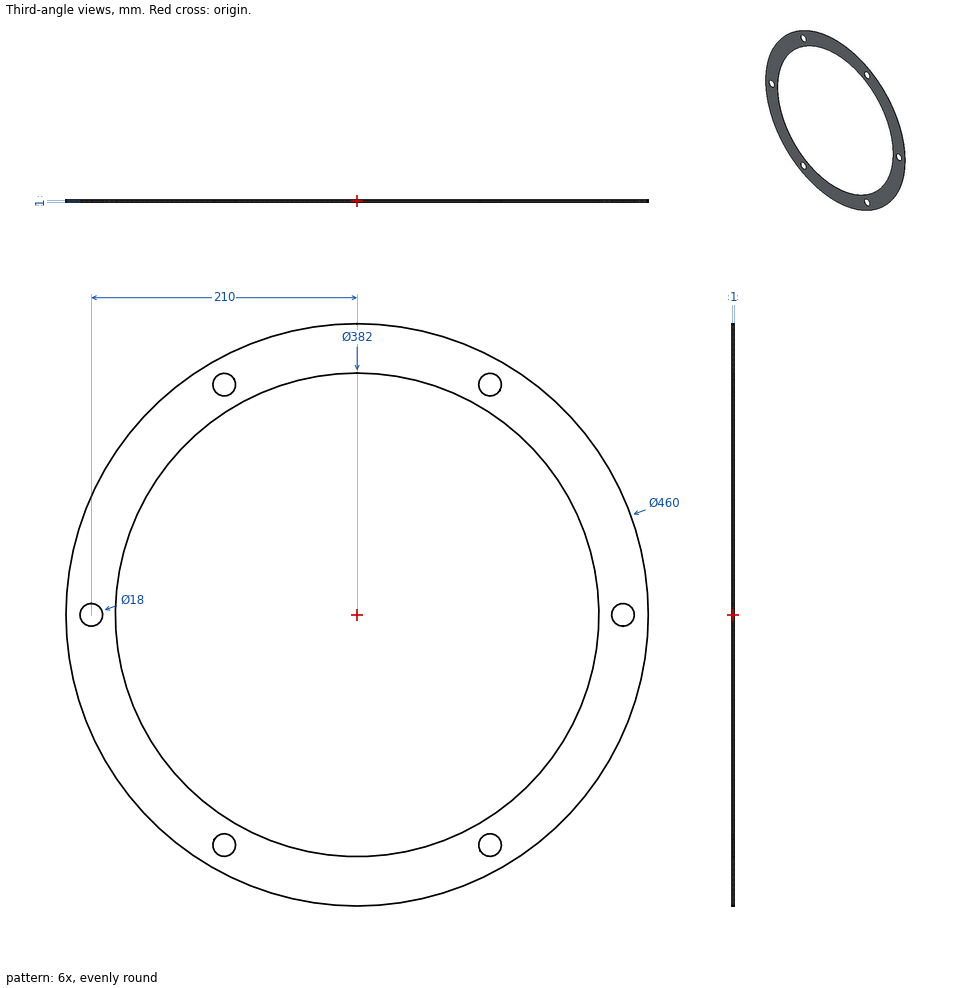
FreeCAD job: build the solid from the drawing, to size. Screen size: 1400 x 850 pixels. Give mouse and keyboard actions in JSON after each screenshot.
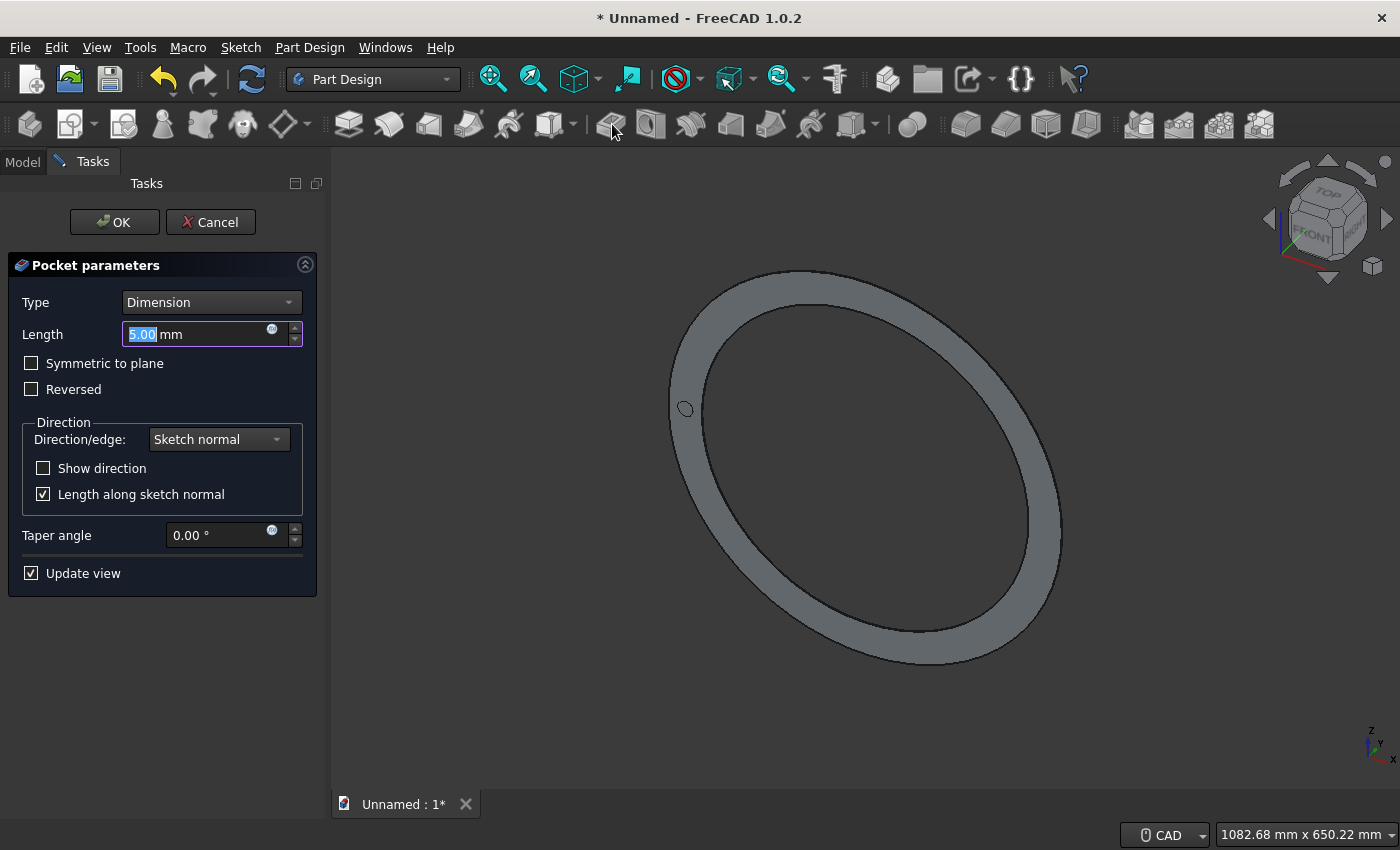
{"action": "type", "text": "1"}
{"action": "key", "text": "Tab"}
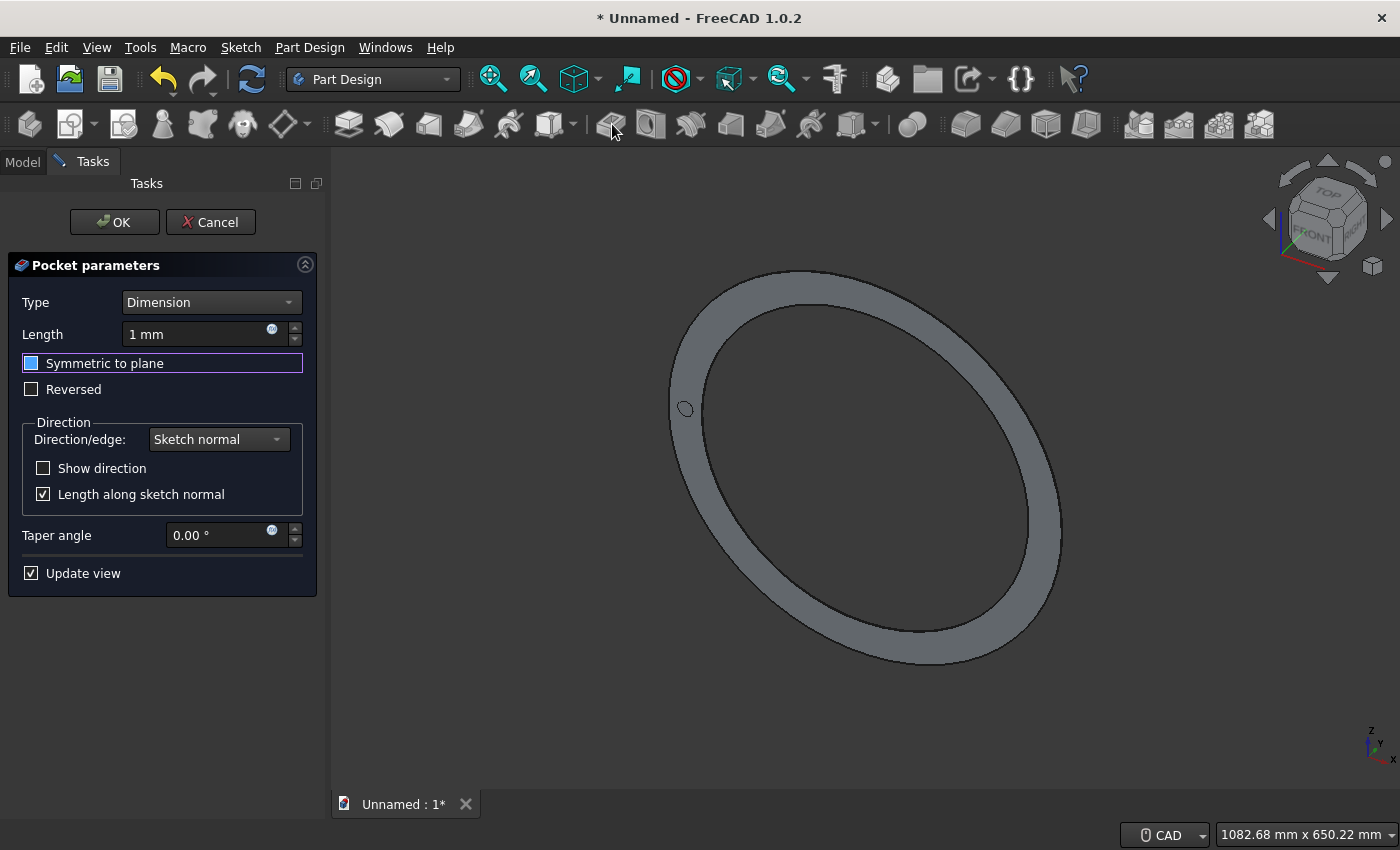
{"action": "left_click", "coordinate": [30, 363]}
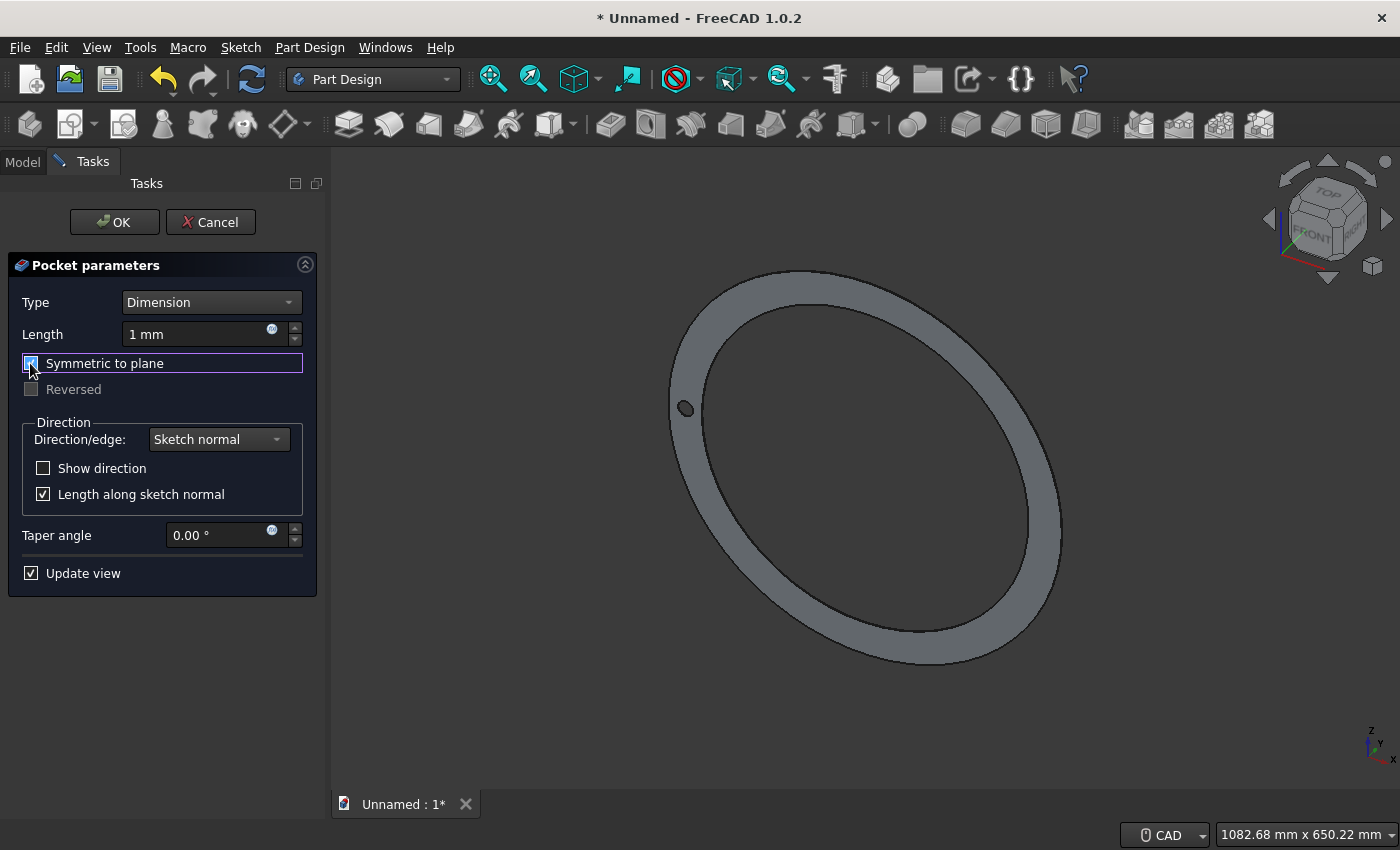
{"action": "left_click", "coordinate": [115, 222]}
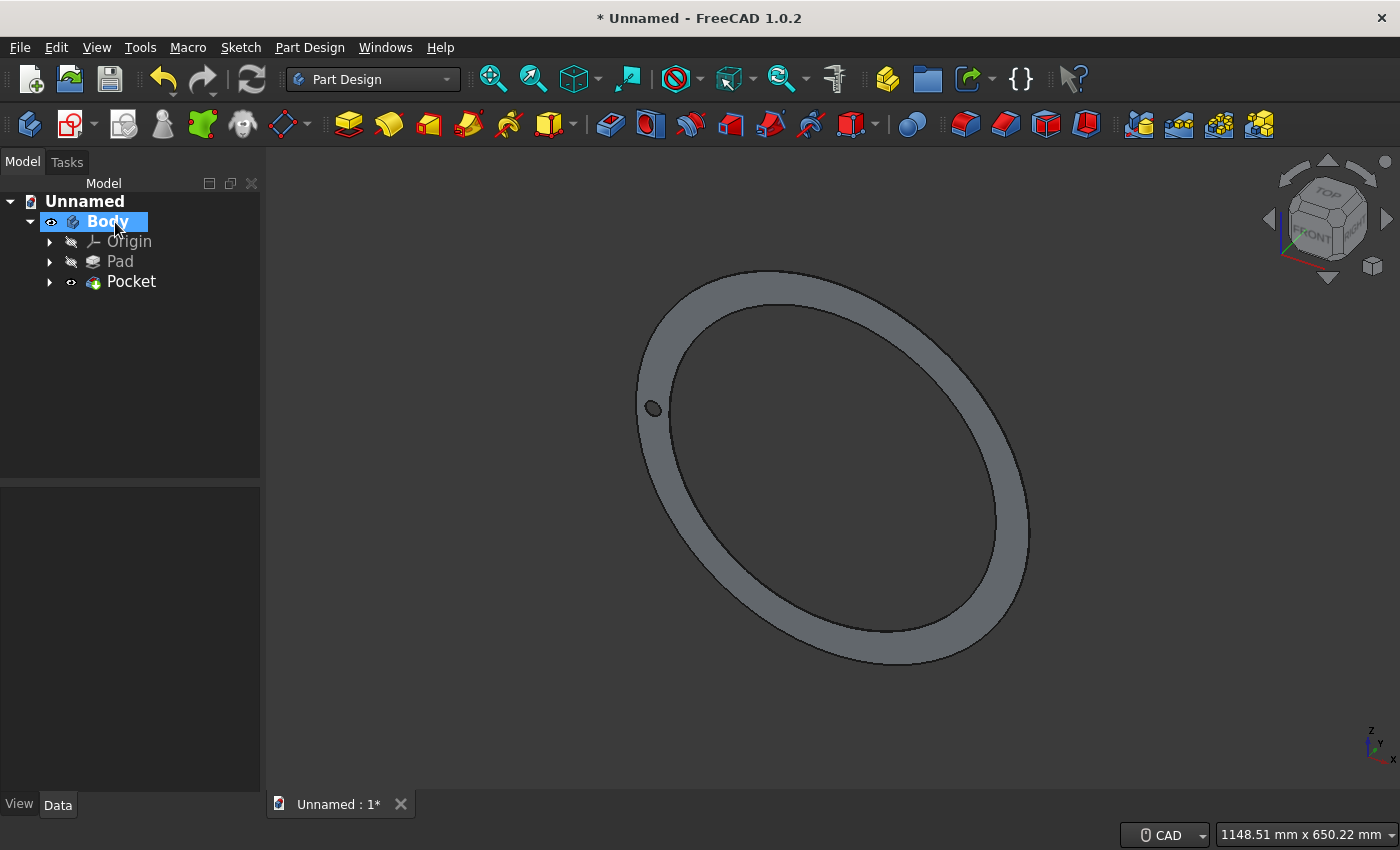
{"action": "left_click", "coordinate": [116, 282]}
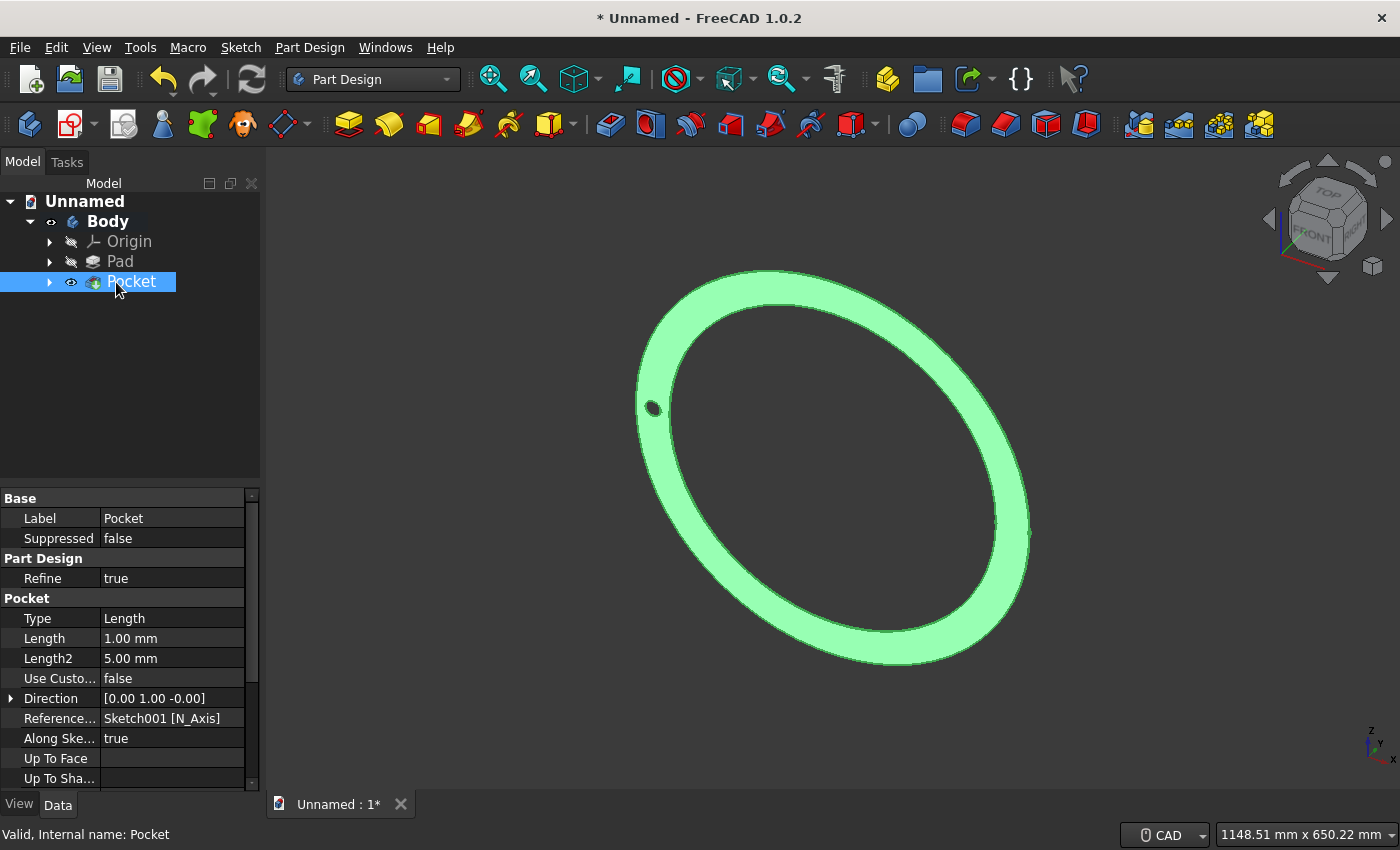
{"action": "left_click", "coordinate": [1220, 124]}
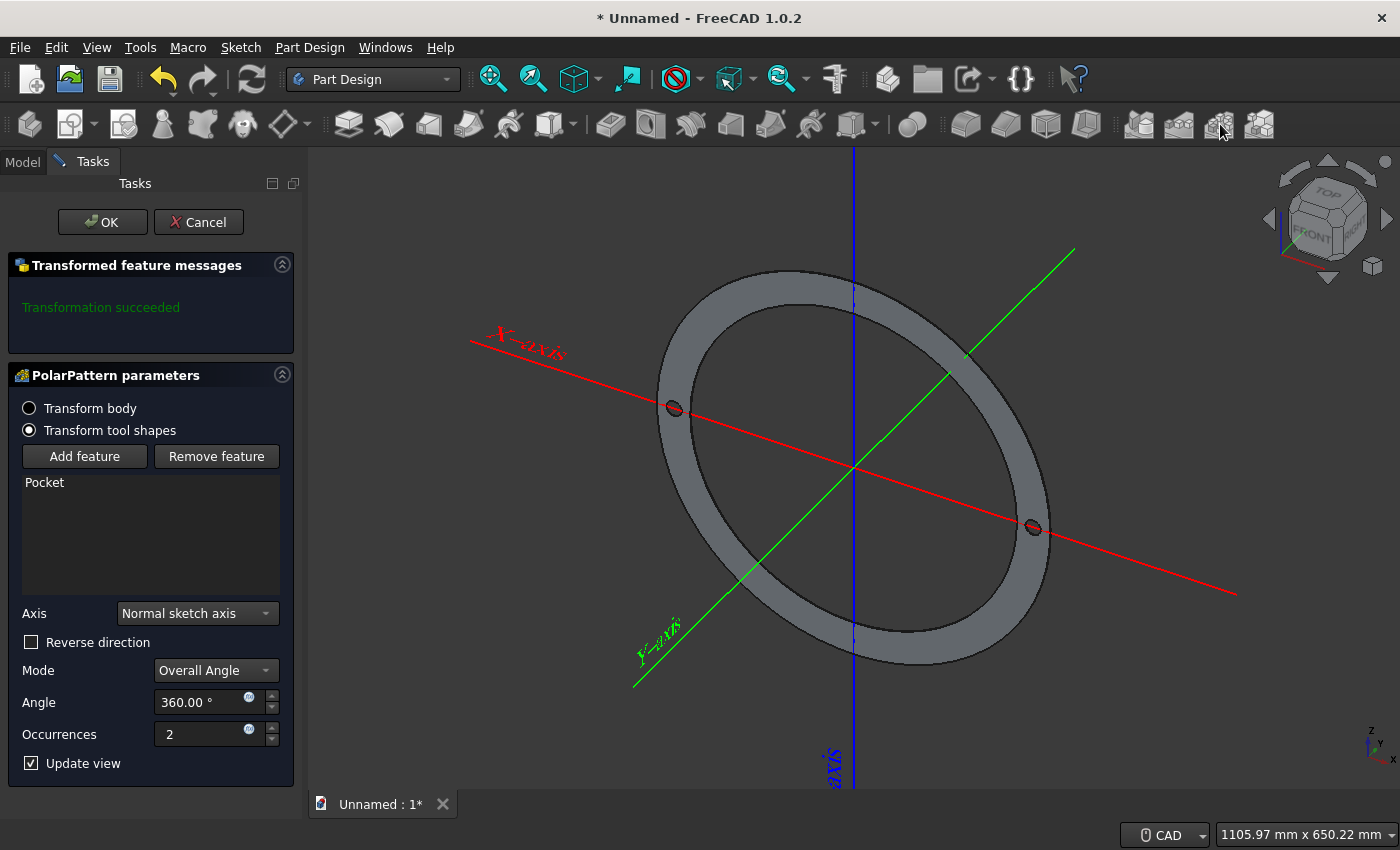
{"action": "left_click", "coordinate": [198, 614]}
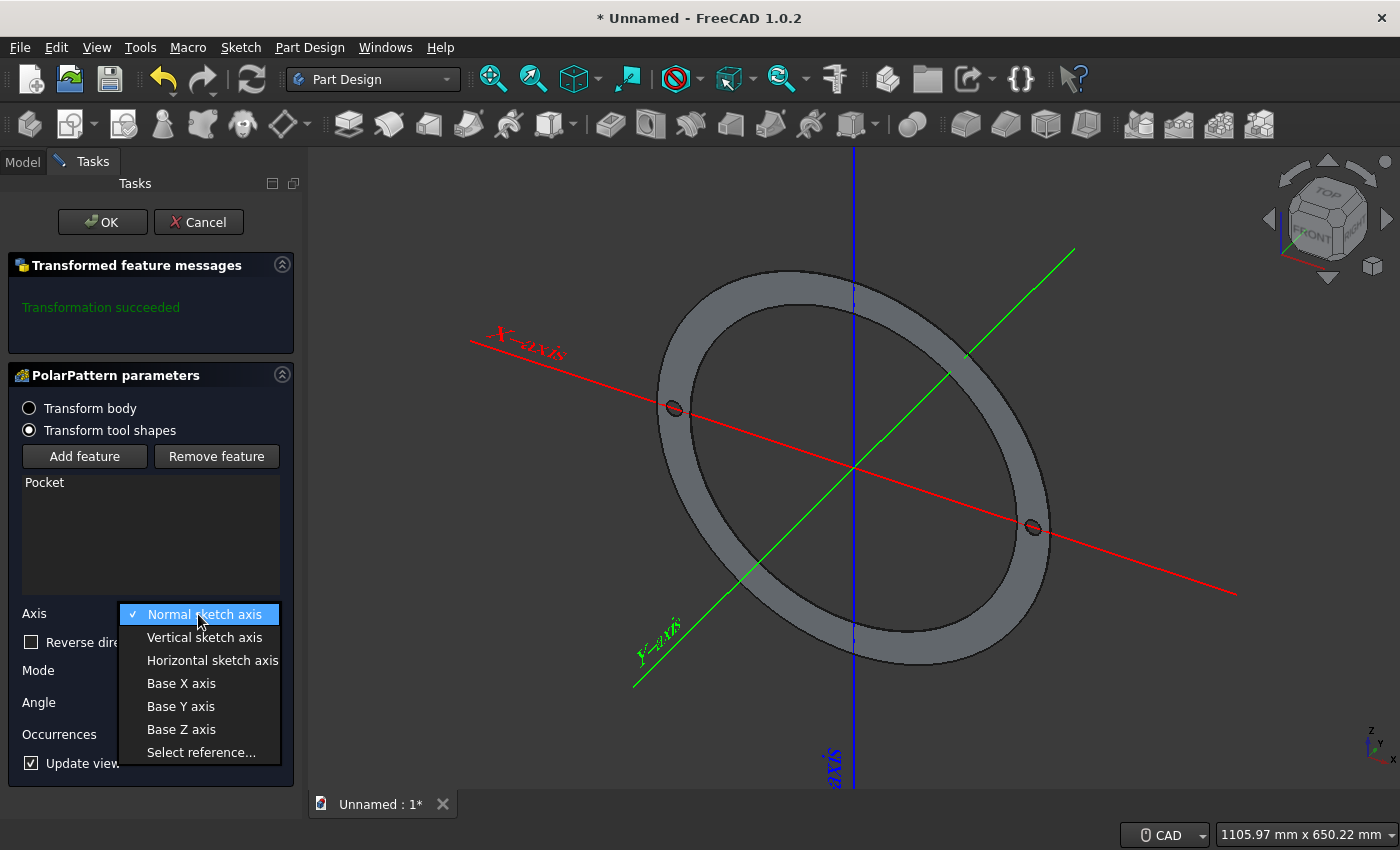
{"action": "left_click", "coordinate": [198, 706]}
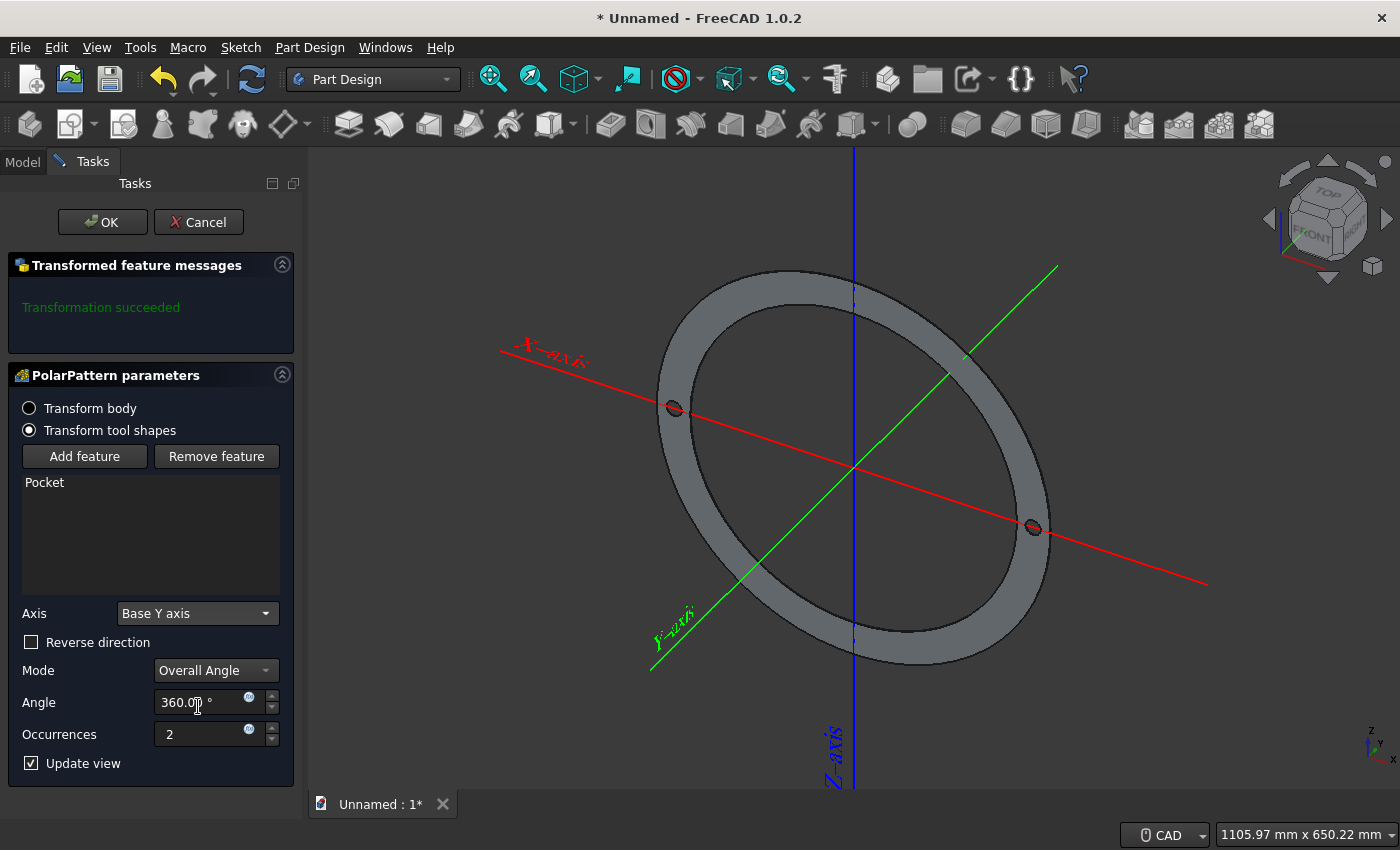
{"action": "triple_click", "coordinate": [209, 734]}